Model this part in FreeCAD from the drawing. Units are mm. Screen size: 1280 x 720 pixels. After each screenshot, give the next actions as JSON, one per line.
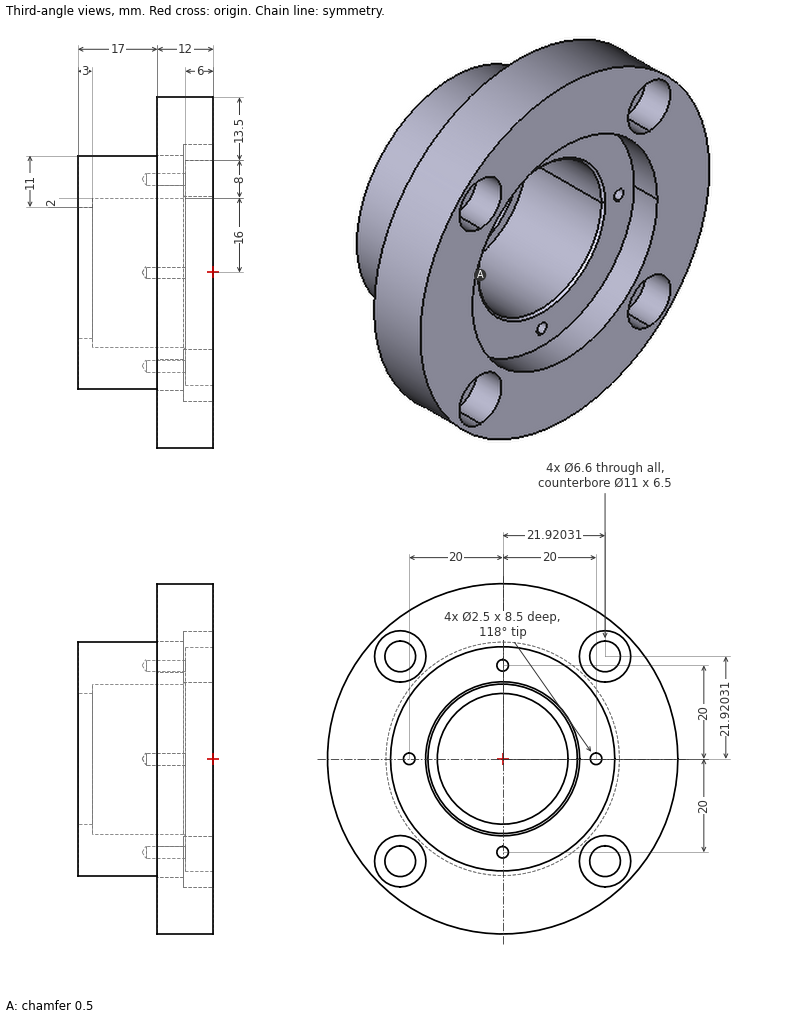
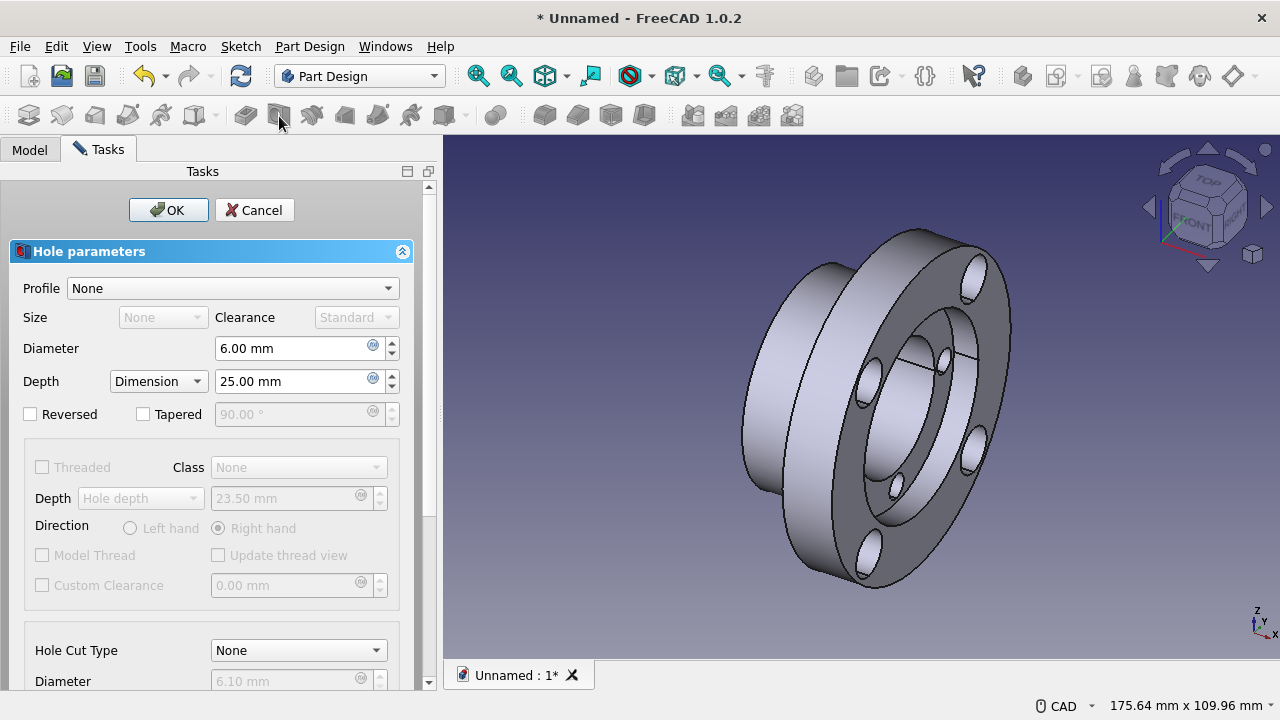
{"action": "triple_click", "coordinate": [300, 348]}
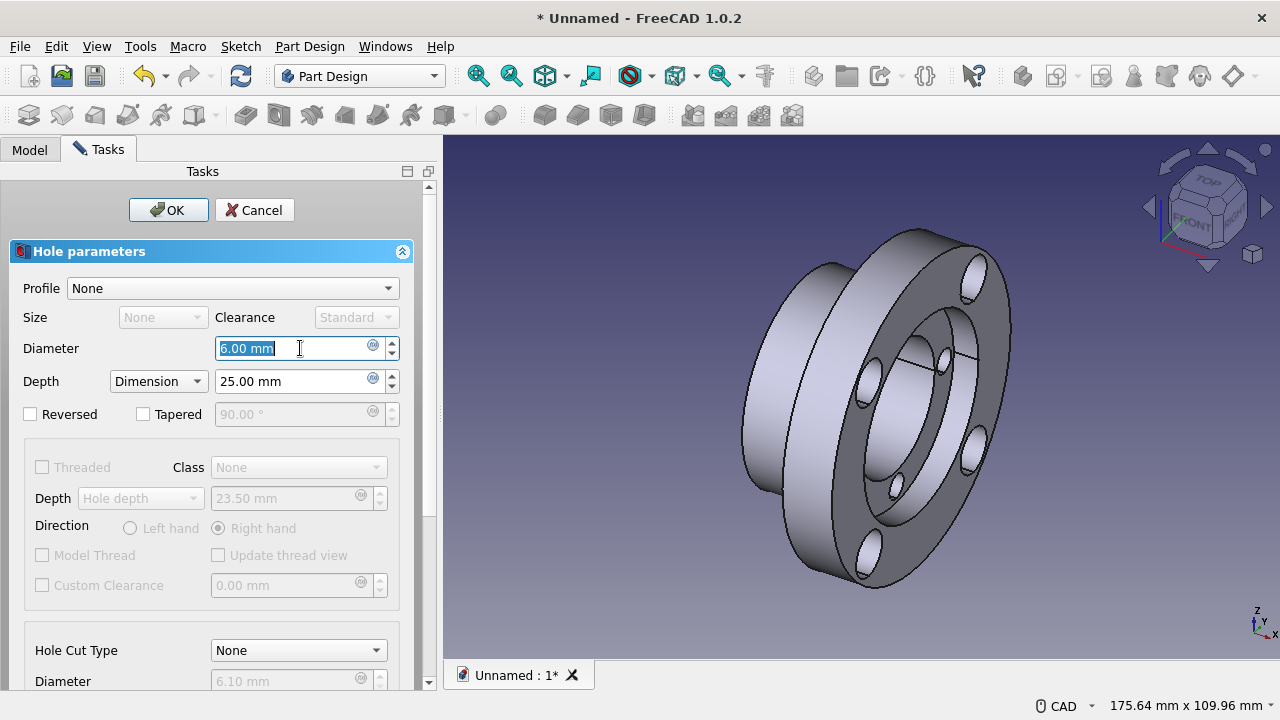
{"action": "type", "text": "2.5"}
{"action": "key", "text": "Tab"}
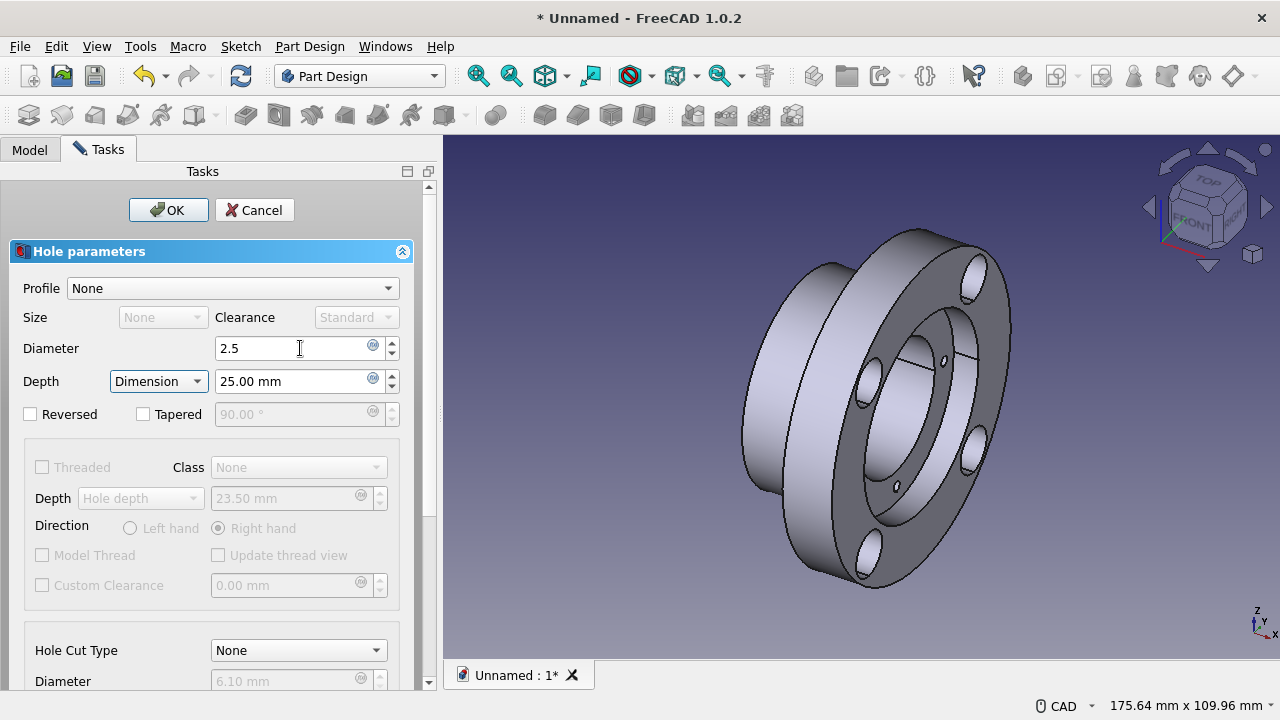
{"action": "triple_click", "coordinate": [300, 382]}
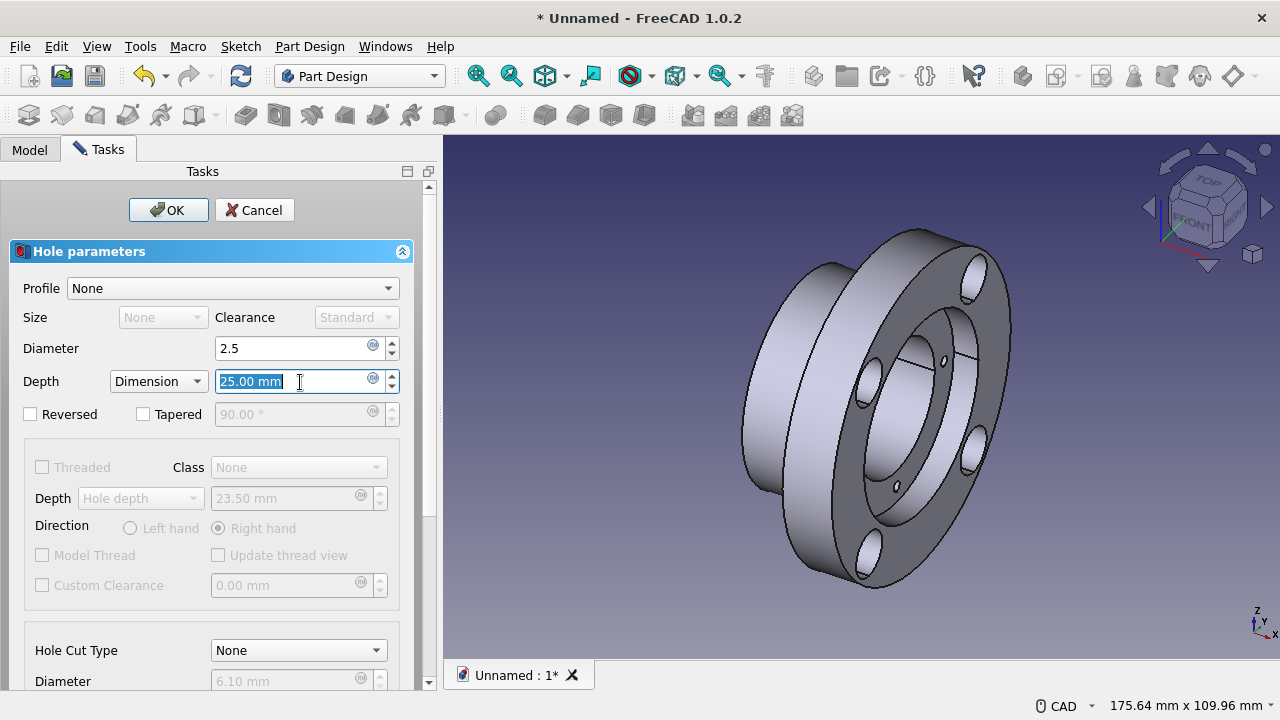
{"action": "type", "text": "8.5"}
{"action": "key", "text": "Tab"}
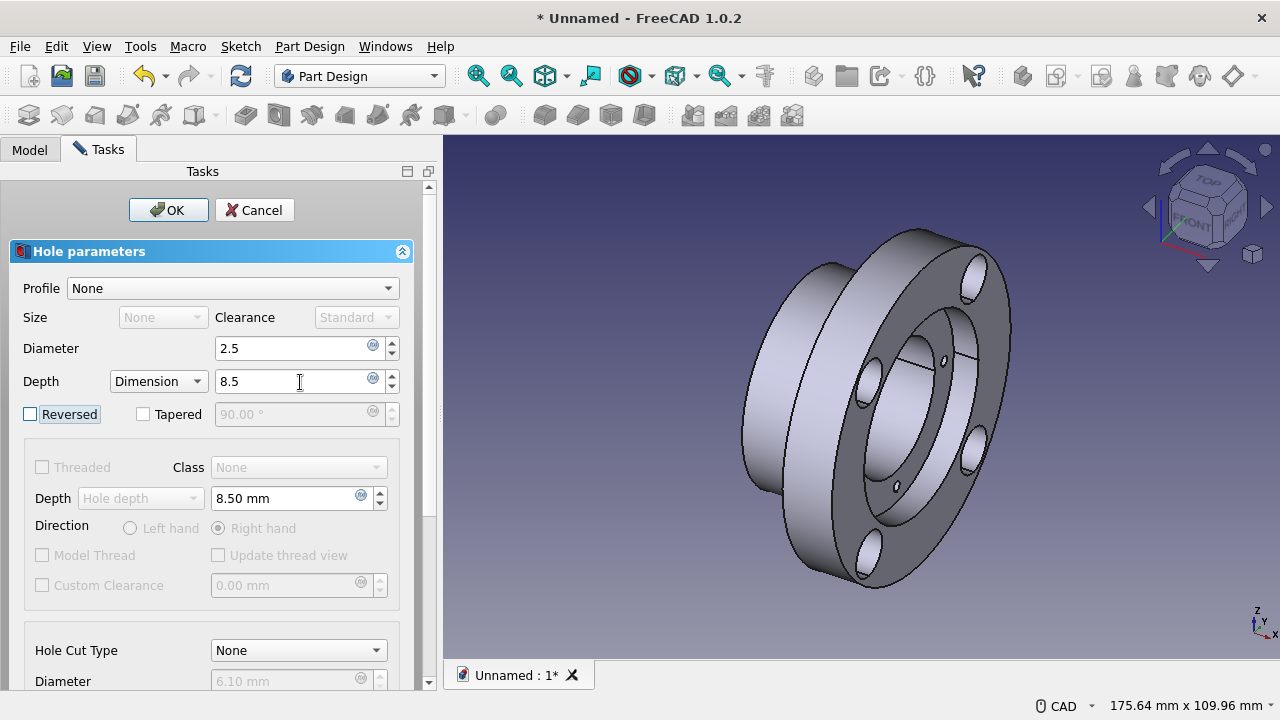
{"action": "left_click", "coordinate": [169, 210]}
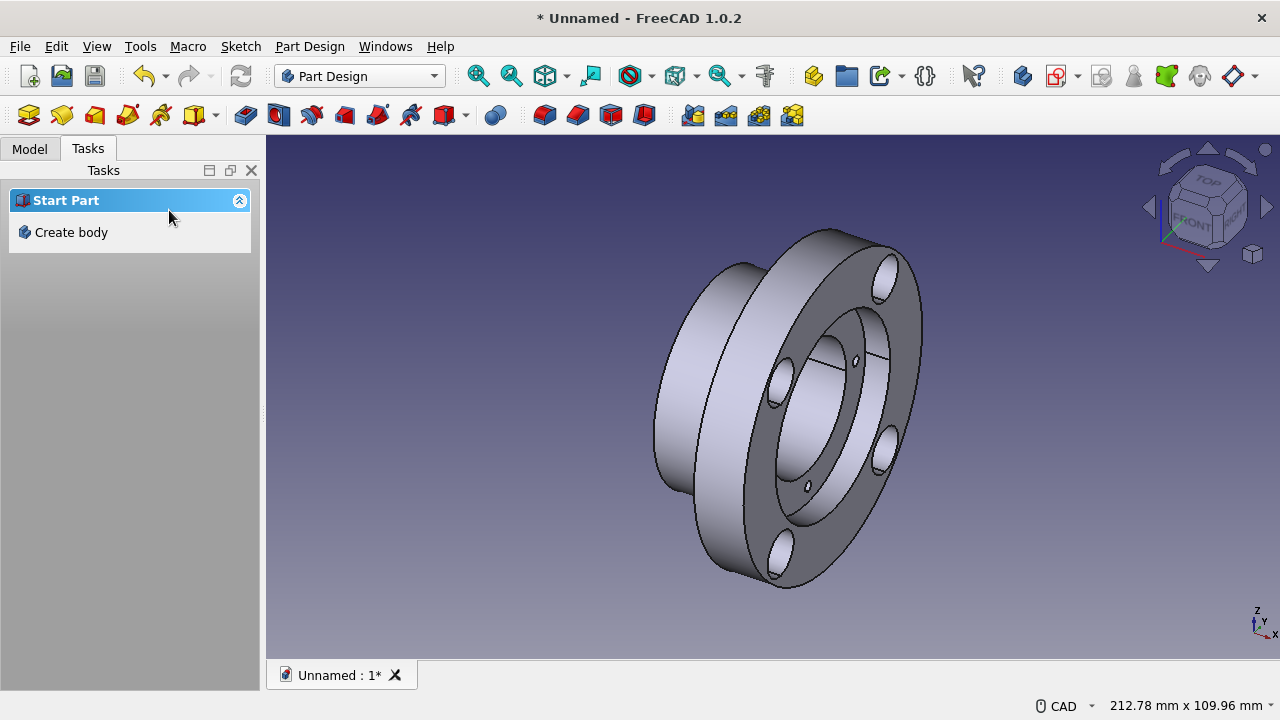
{"action": "left_click", "coordinate": [796, 479]}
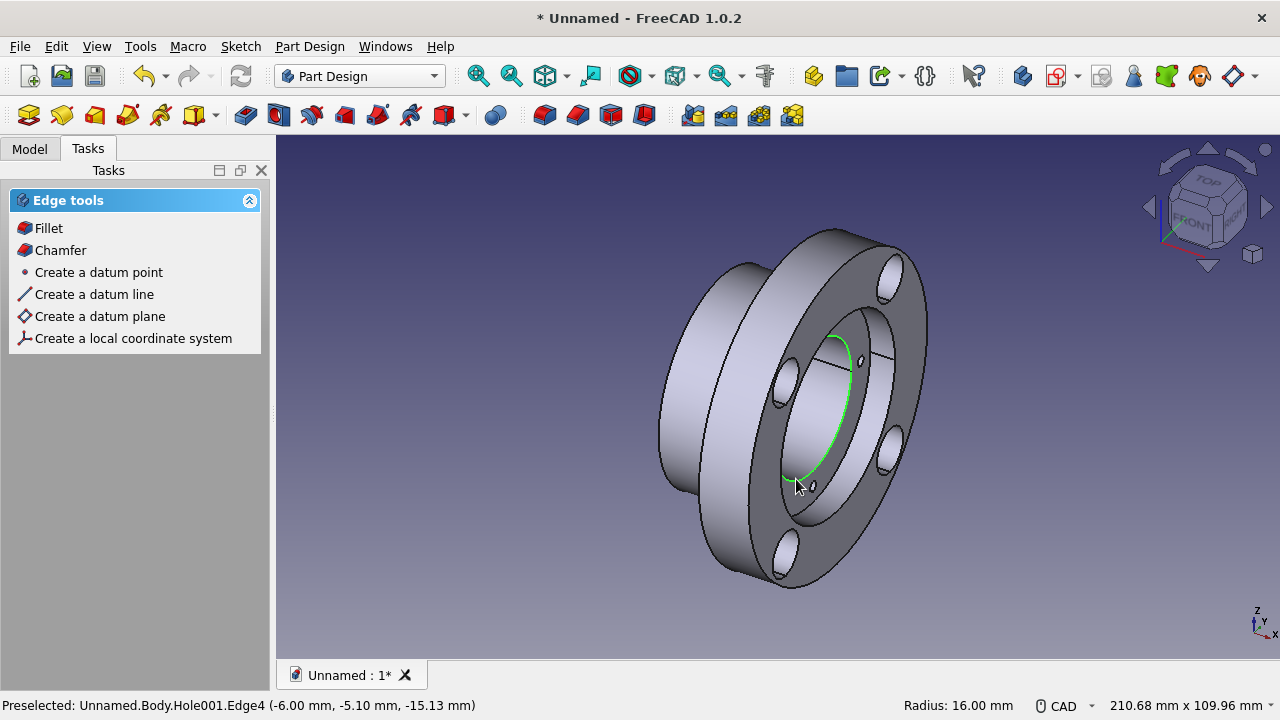
{"action": "left_click", "coordinate": [578, 116]}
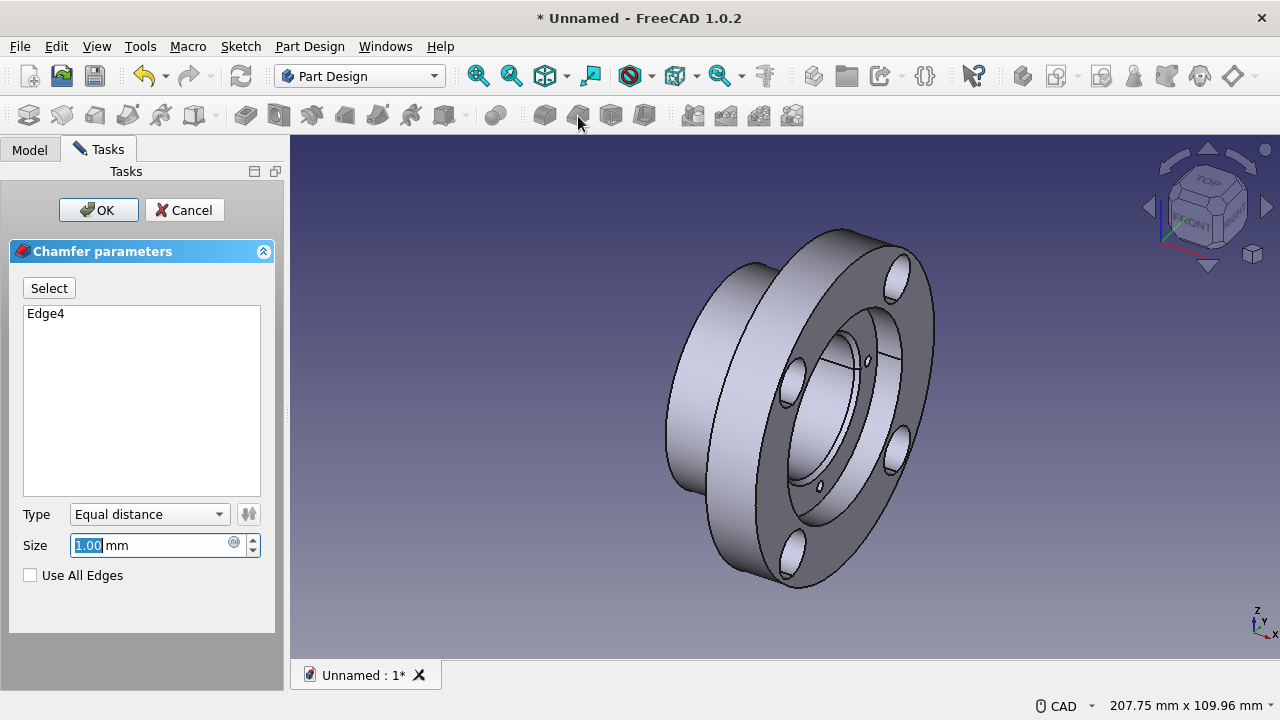
{"action": "type", "text": "0.5"}
{"action": "key", "text": "Tab"}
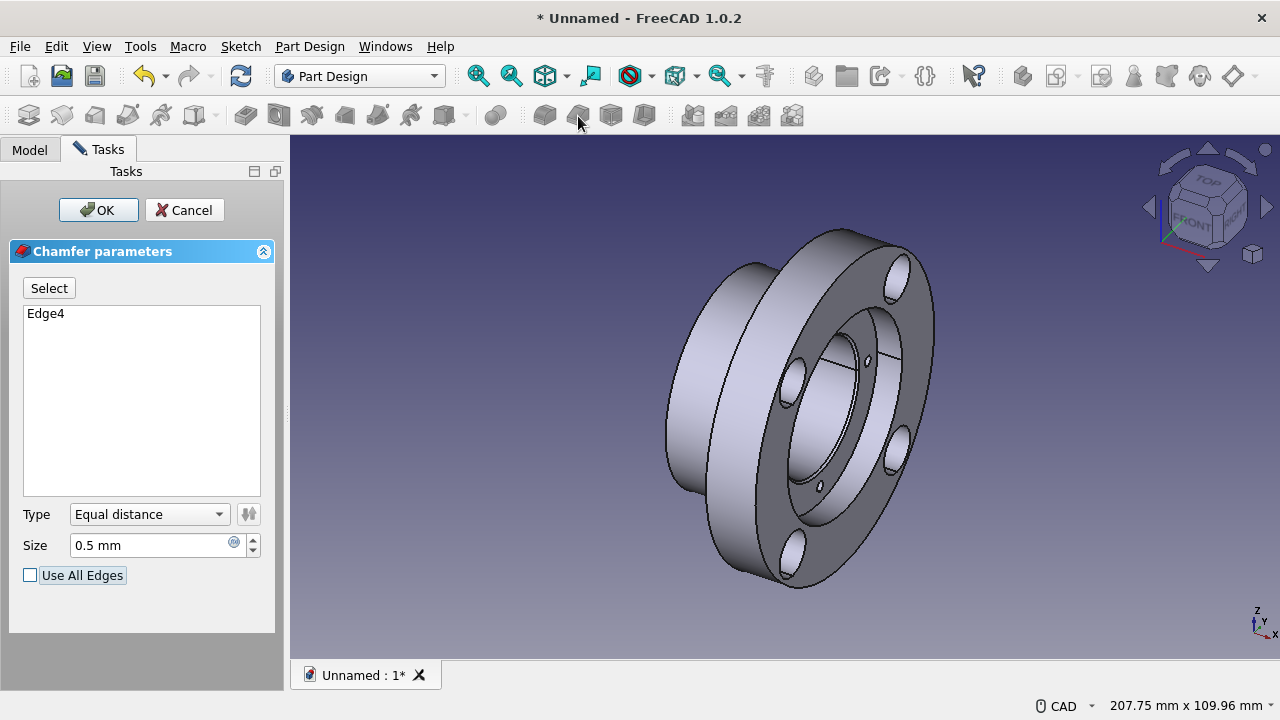
{"action": "left_click", "coordinate": [99, 210]}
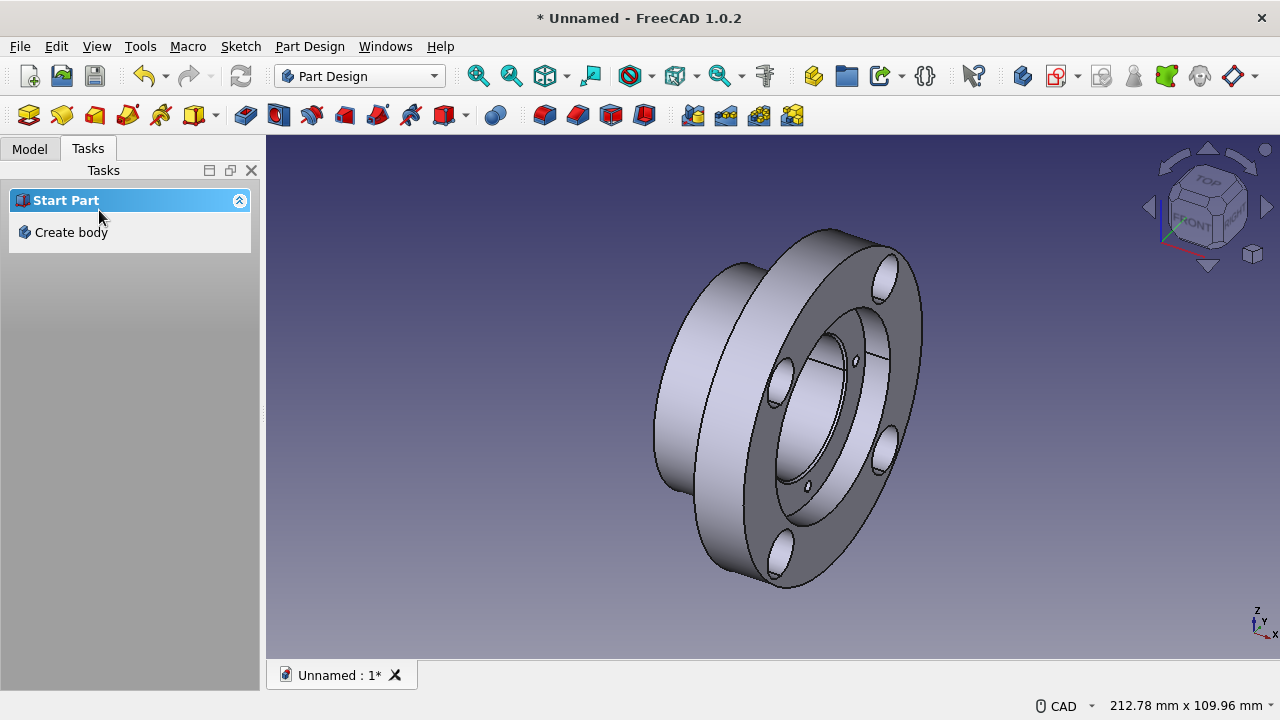
{"action": "key", "text": "0"}